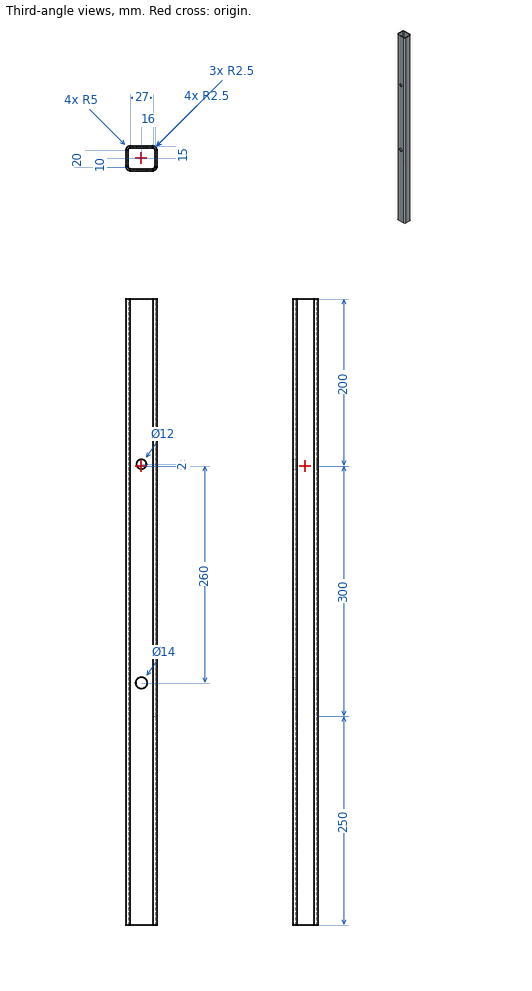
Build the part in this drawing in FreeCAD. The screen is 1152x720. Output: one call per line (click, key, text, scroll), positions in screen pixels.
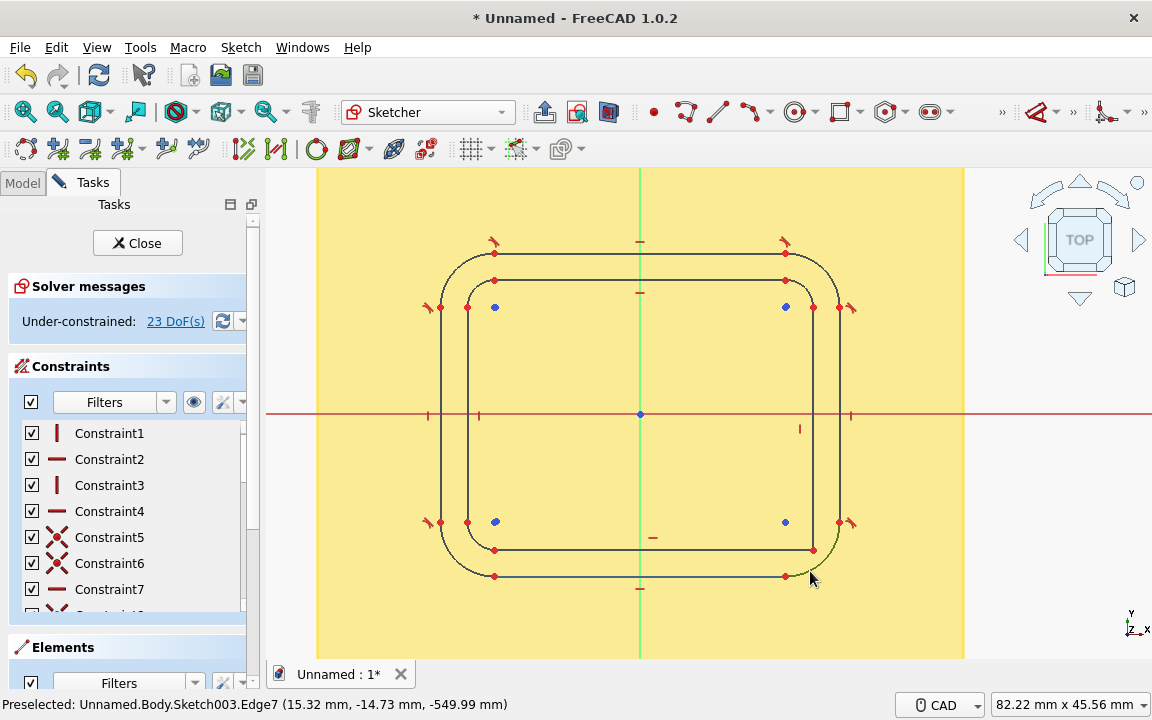
key(t)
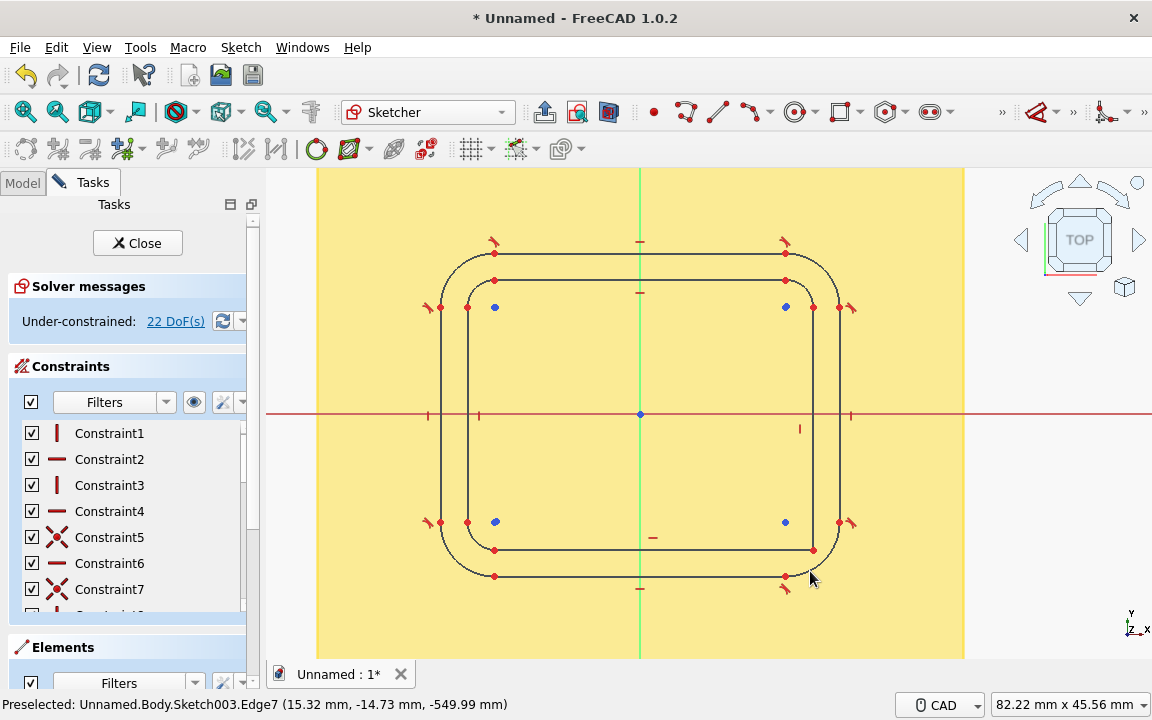
click(698, 577)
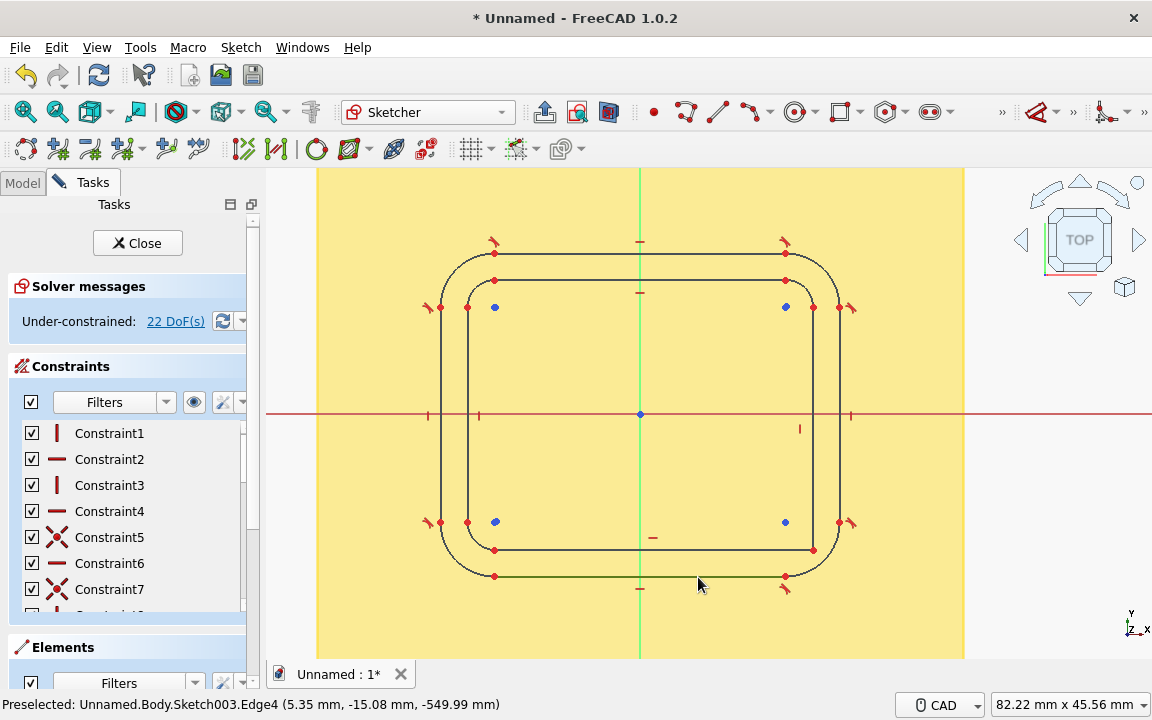
click(446, 547)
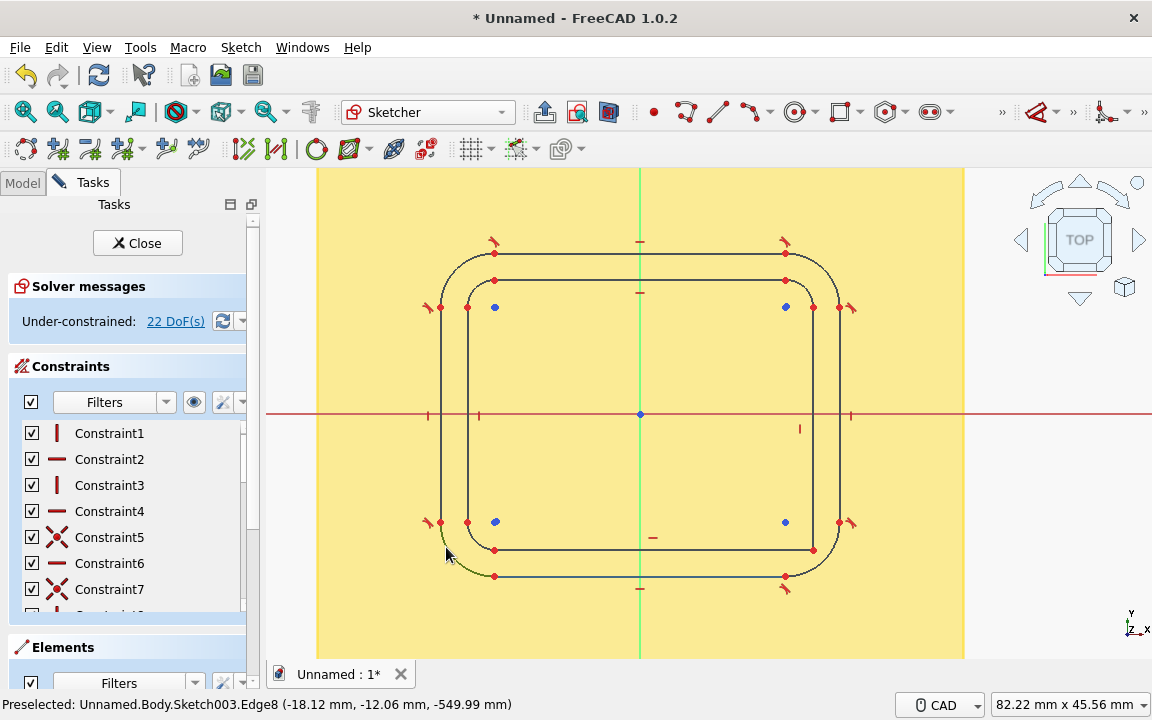
key(t)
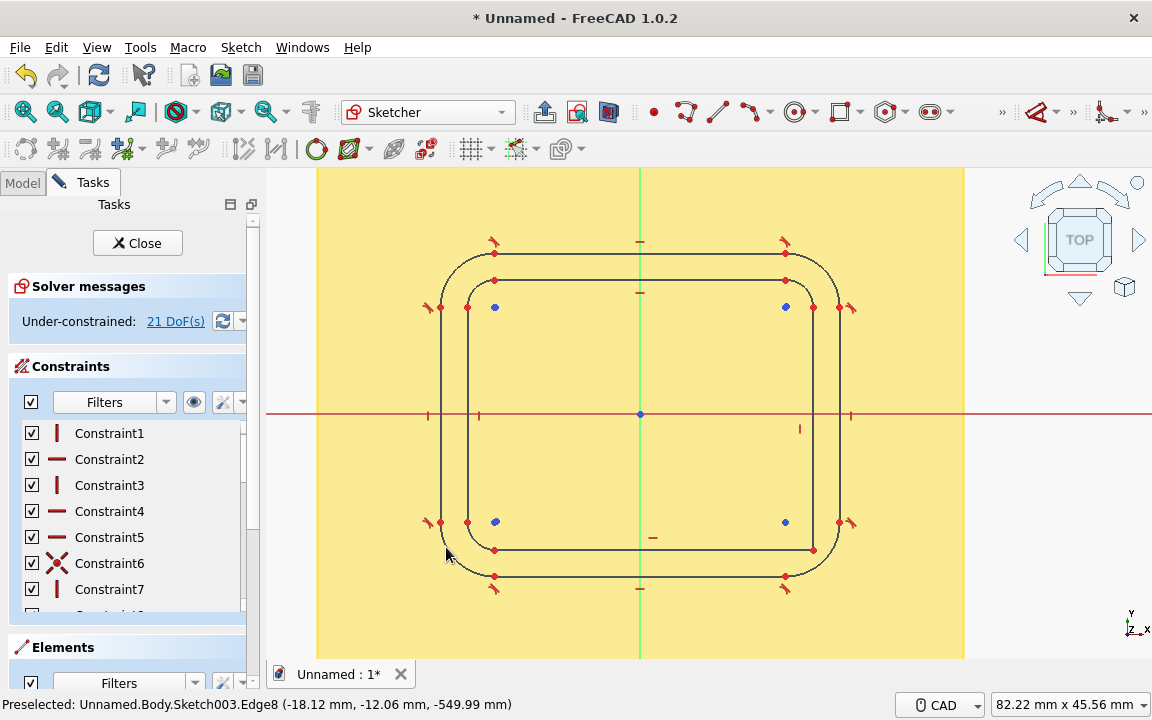
click(590, 550)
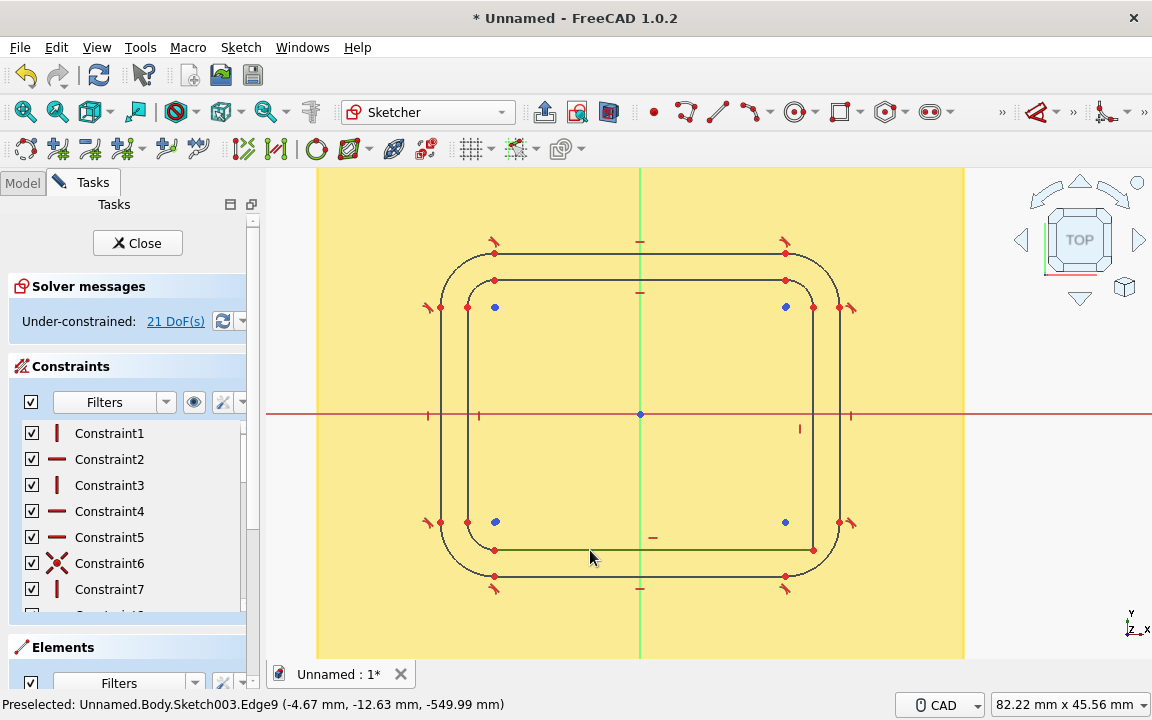
click(471, 535)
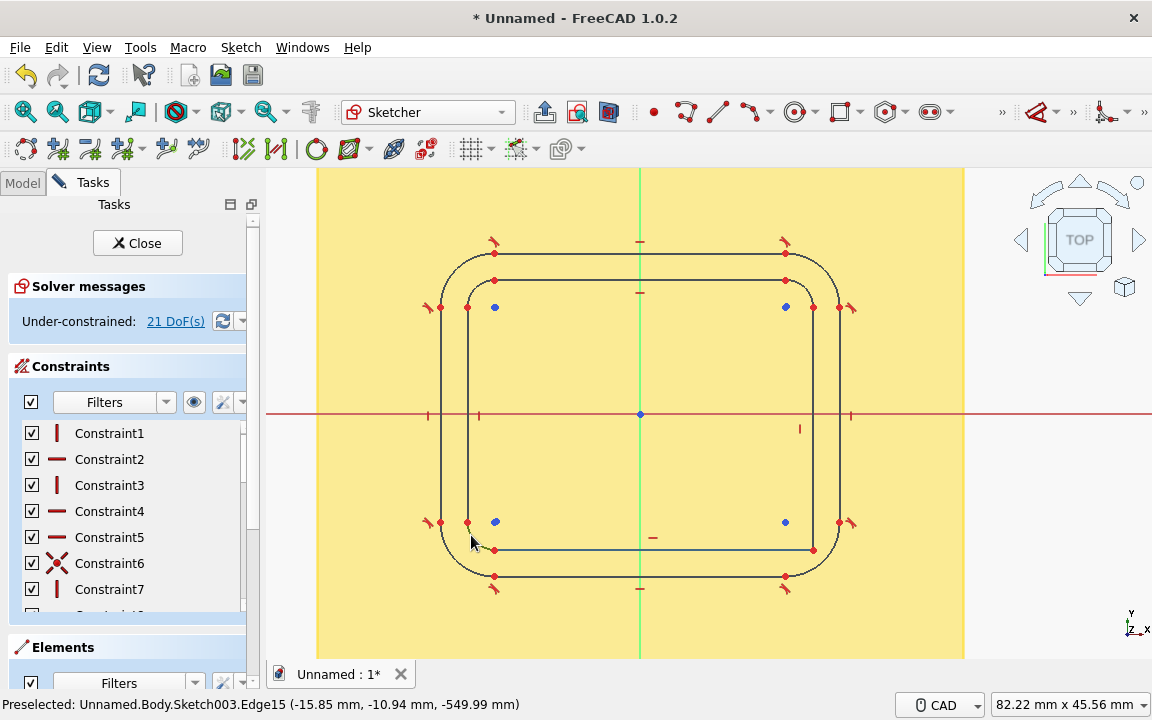
key(t)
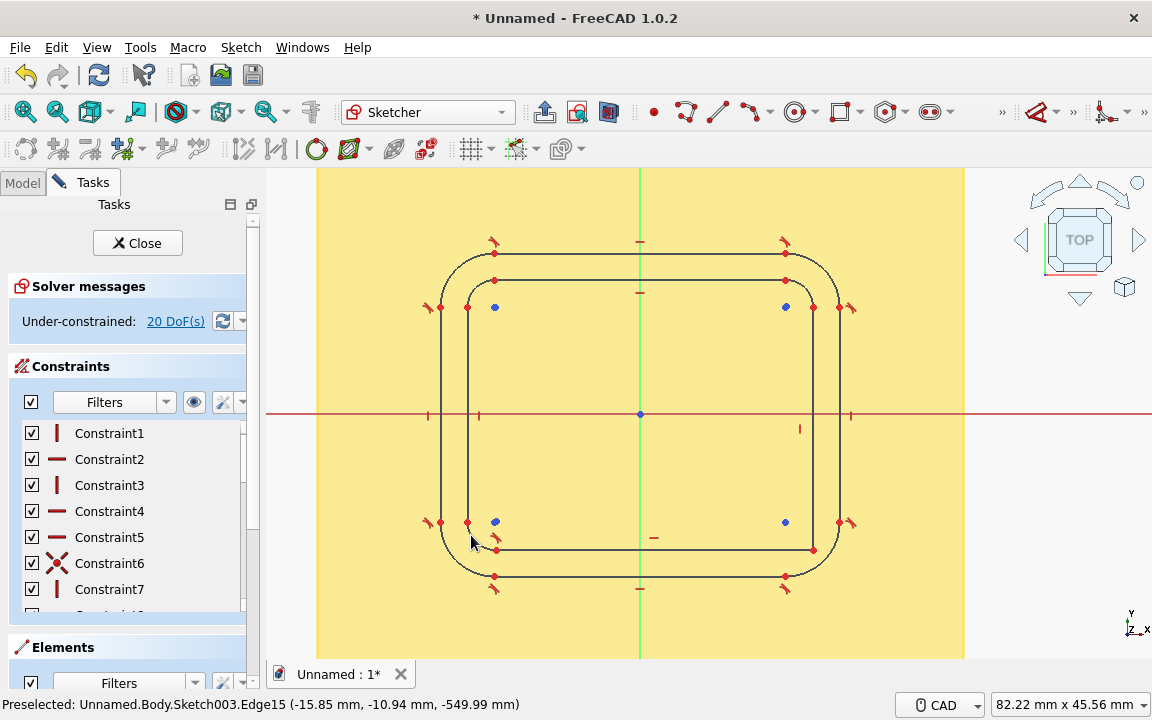
click(813, 477)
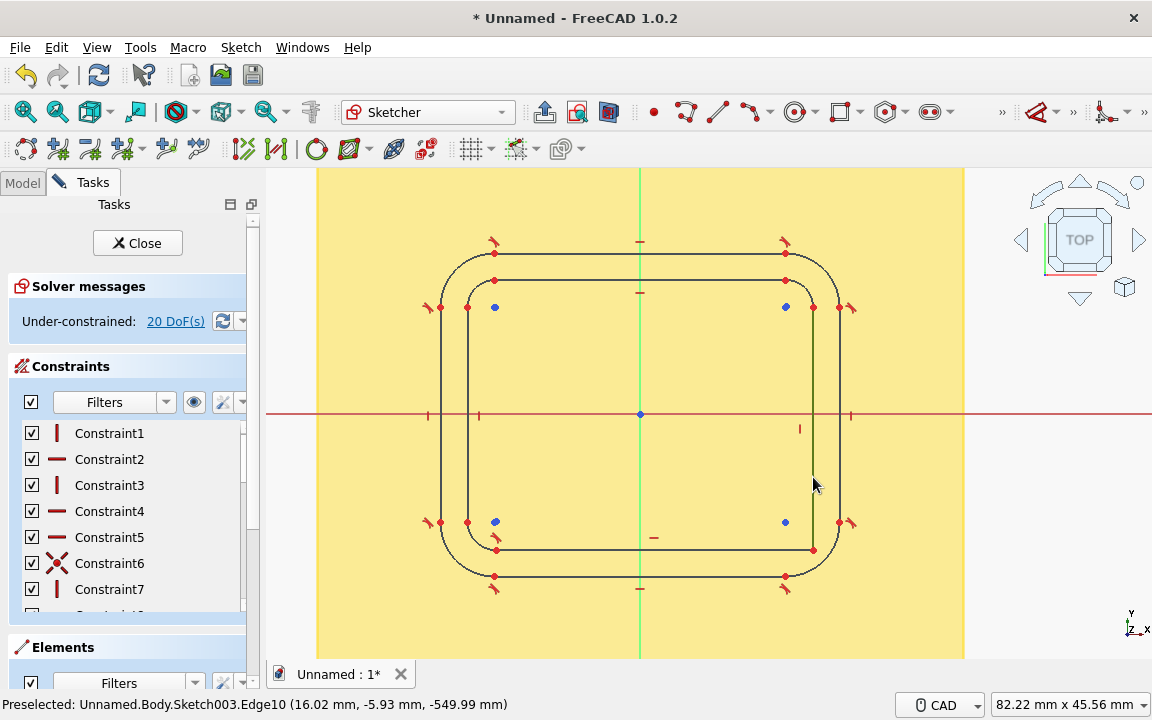
click(810, 295)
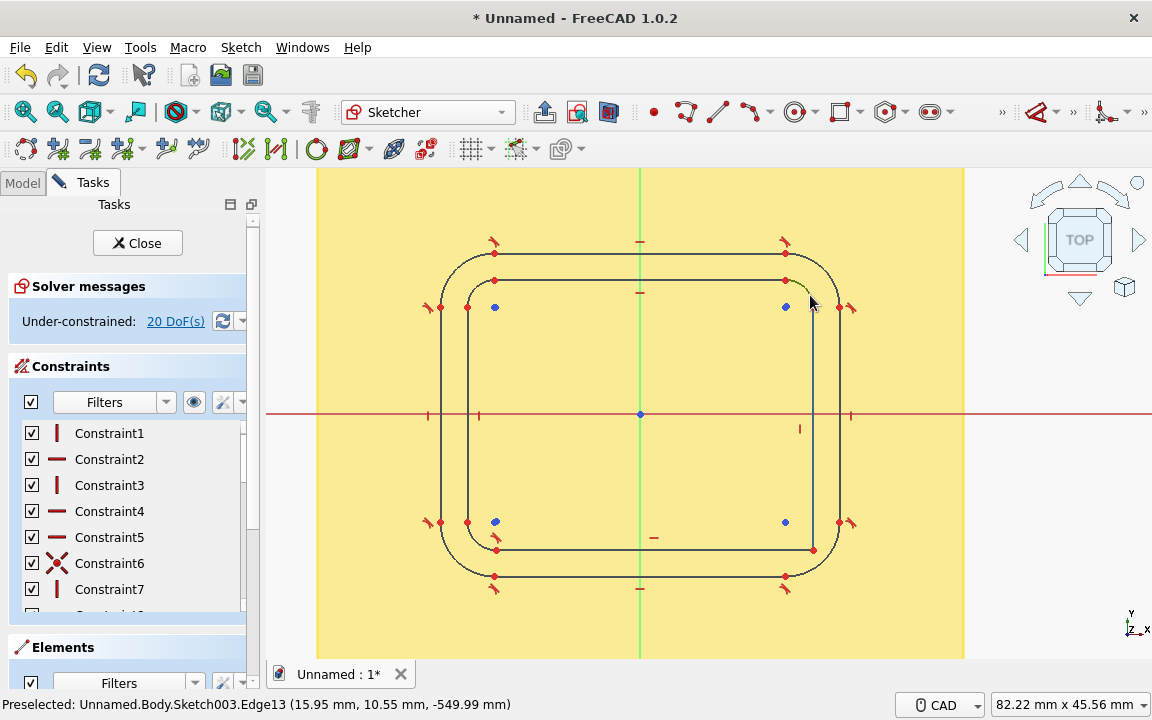
key(t)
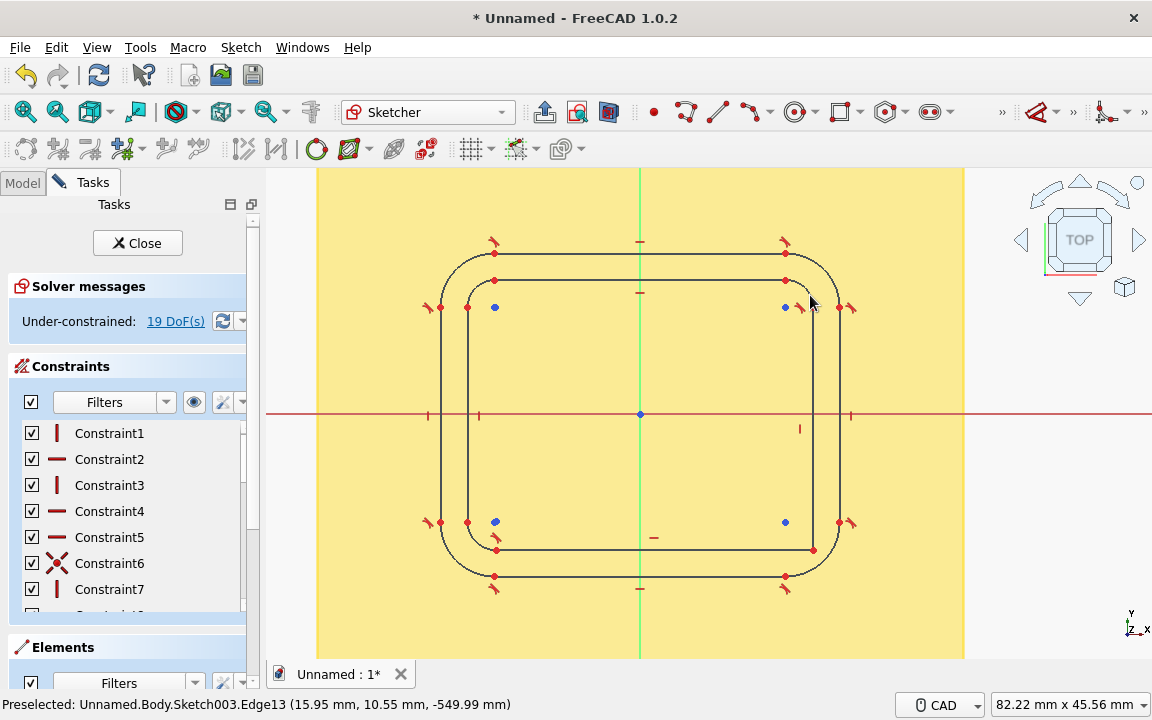
click(699, 280)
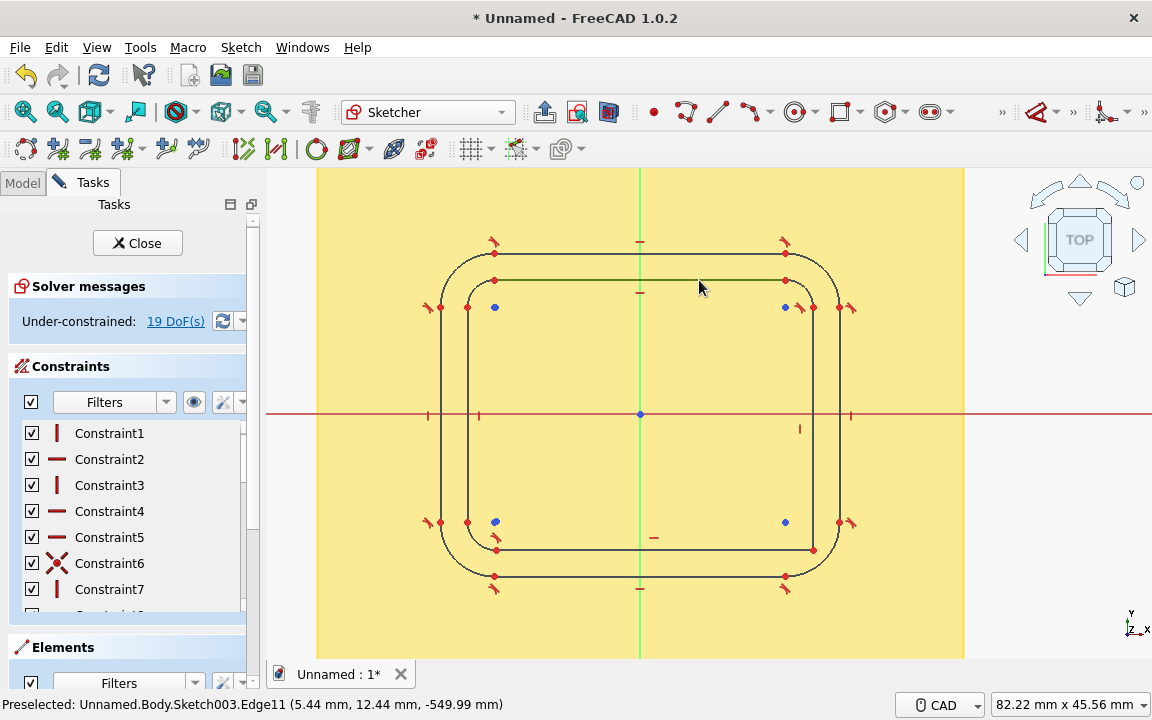
click(810, 295)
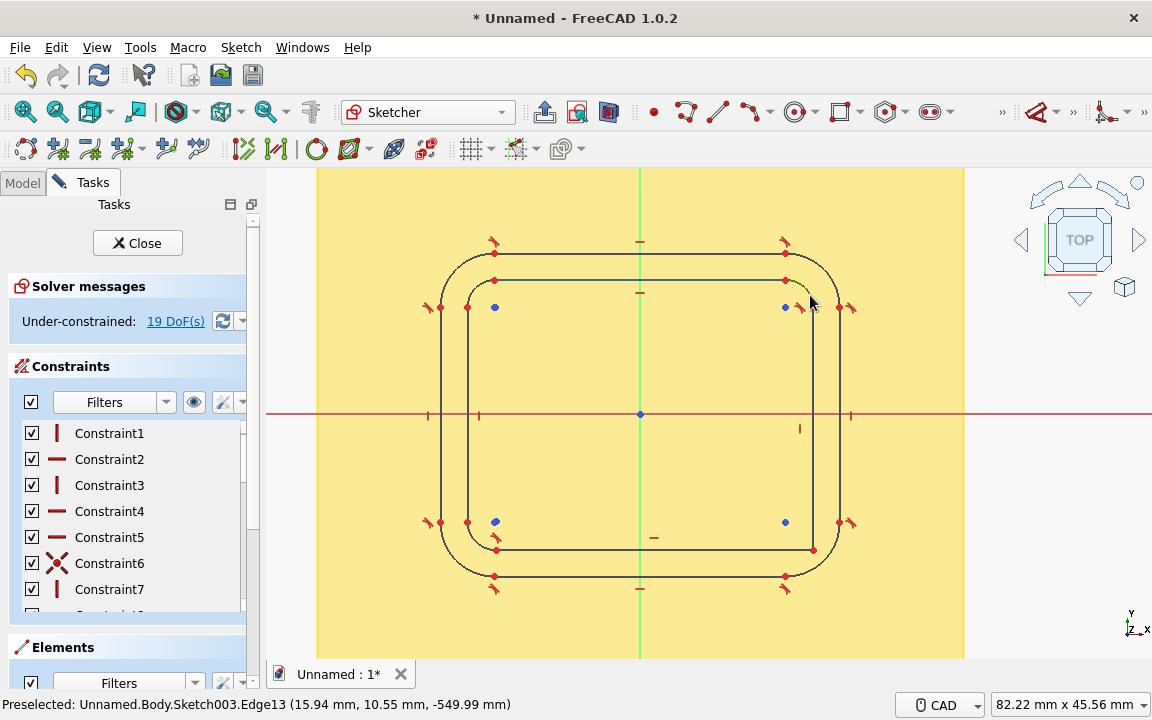
key(t)